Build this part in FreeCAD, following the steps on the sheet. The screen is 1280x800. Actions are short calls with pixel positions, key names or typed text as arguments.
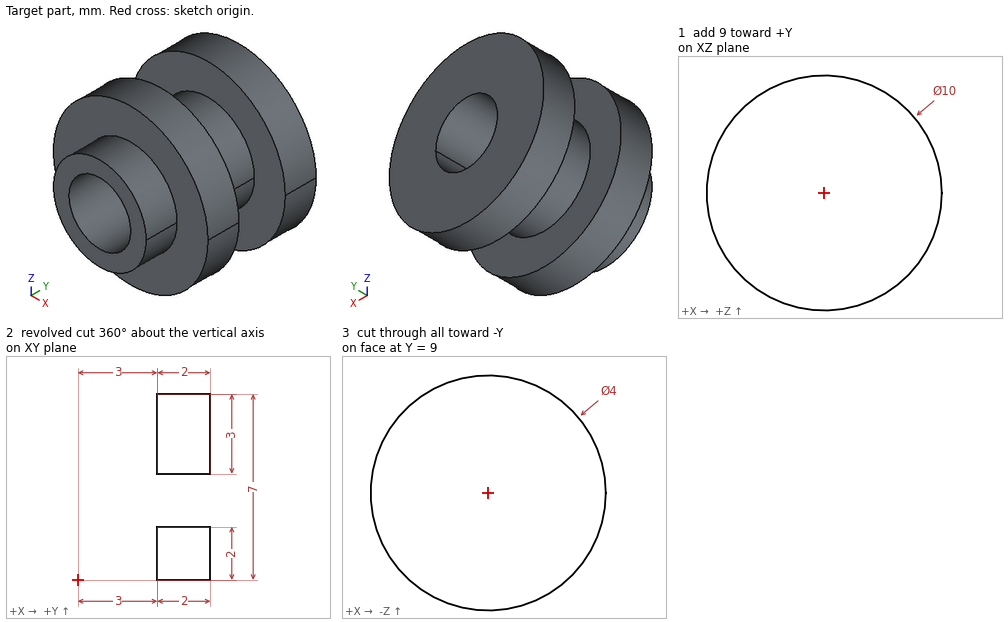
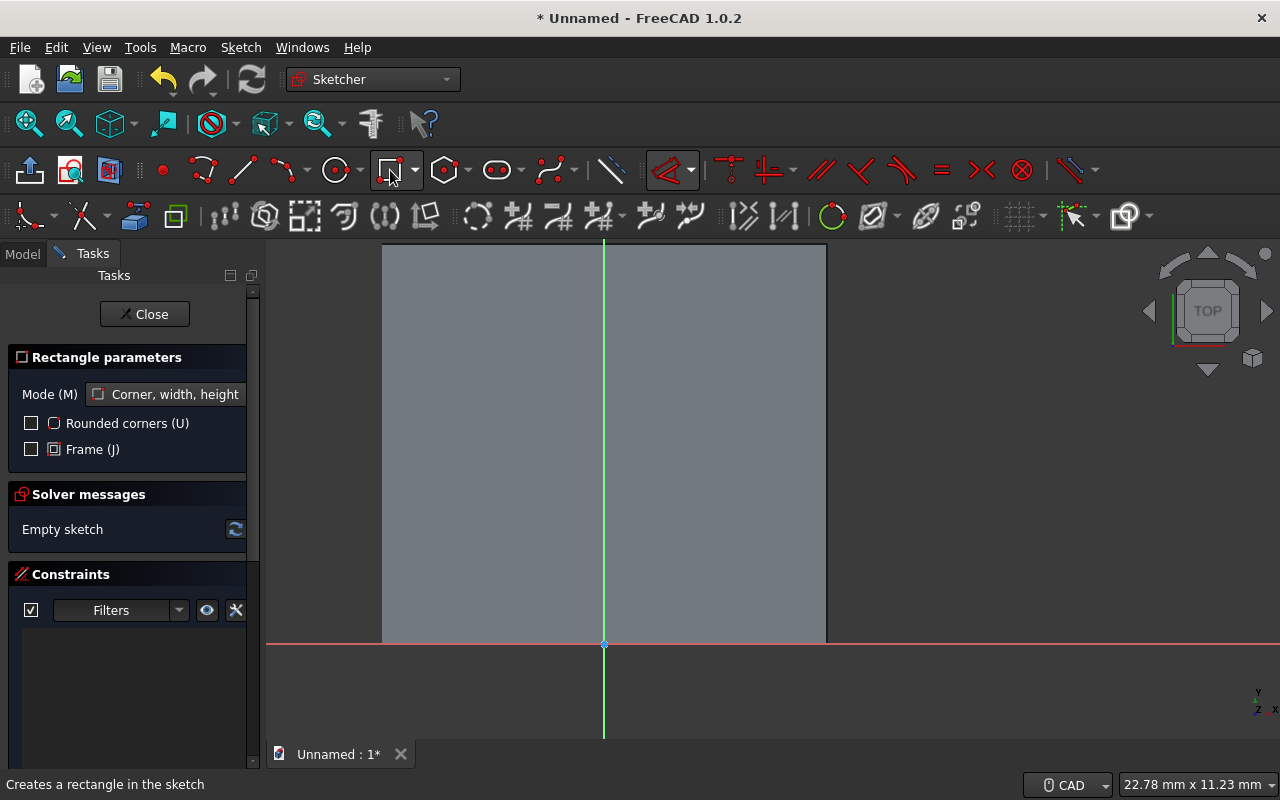
click(738, 333)
move(827, 466)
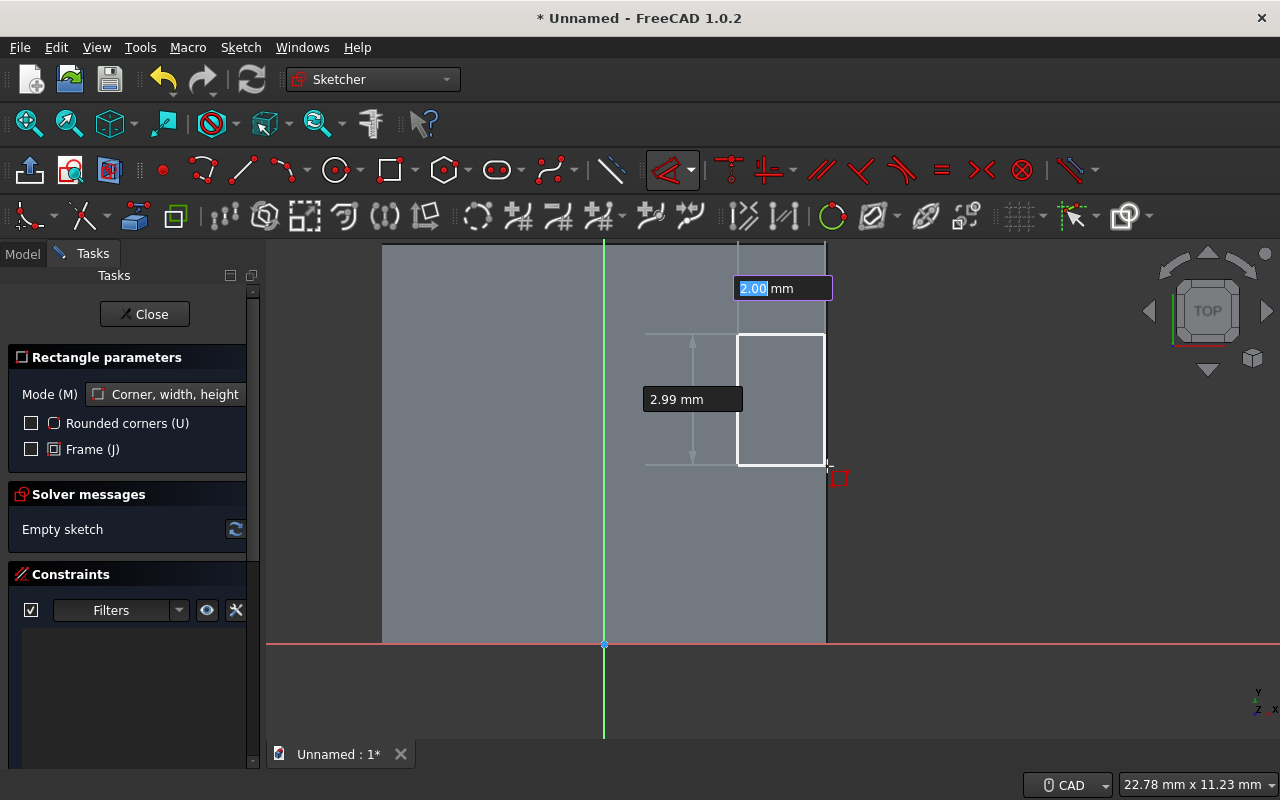
text(2)
key(Tab)
text(3)
key(Return)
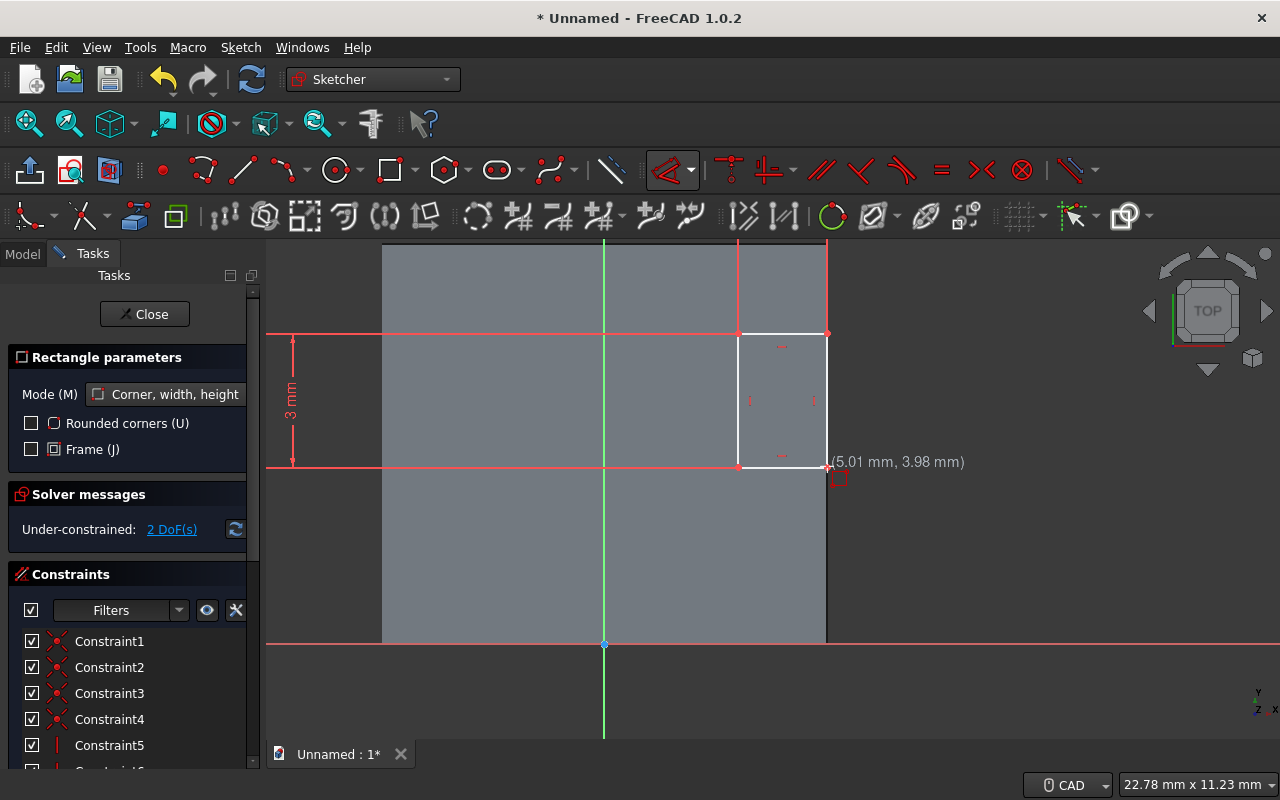
click(738, 555)
click(827, 644)
key(Escape)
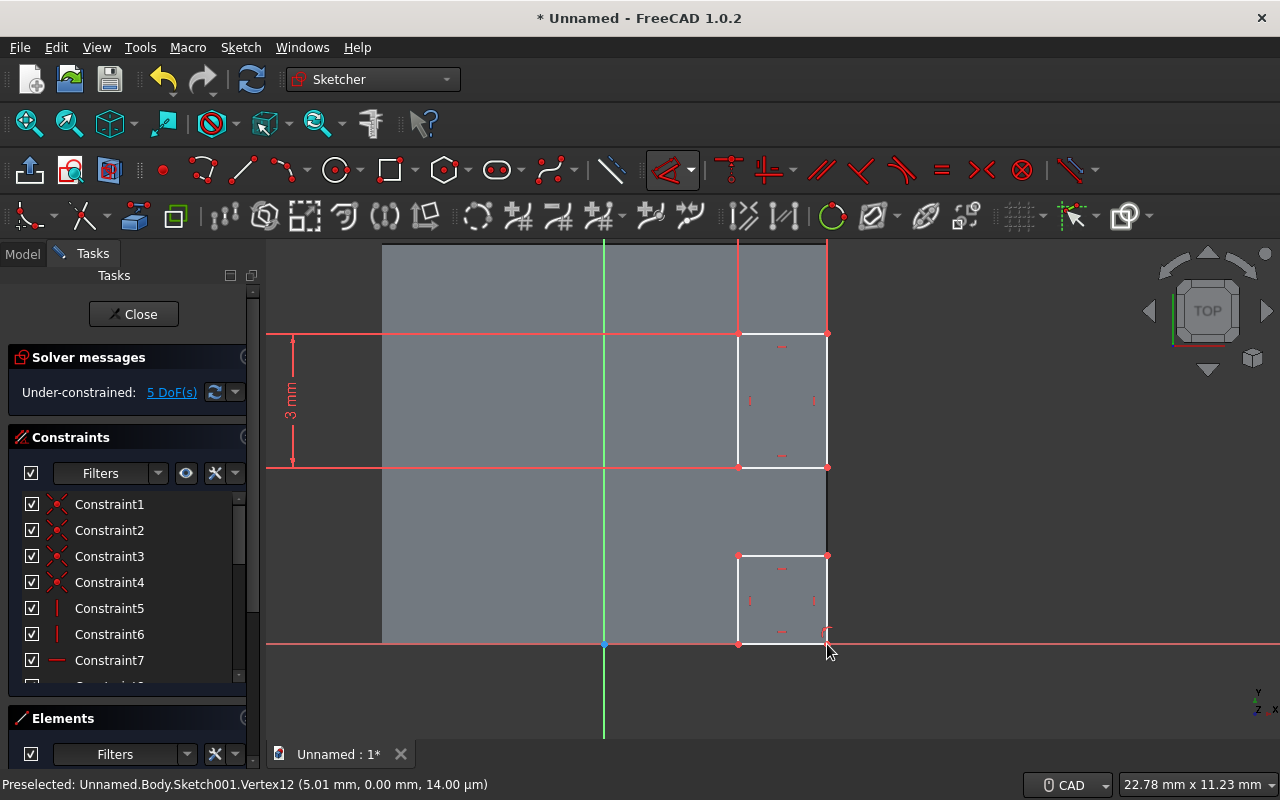
click(738, 582)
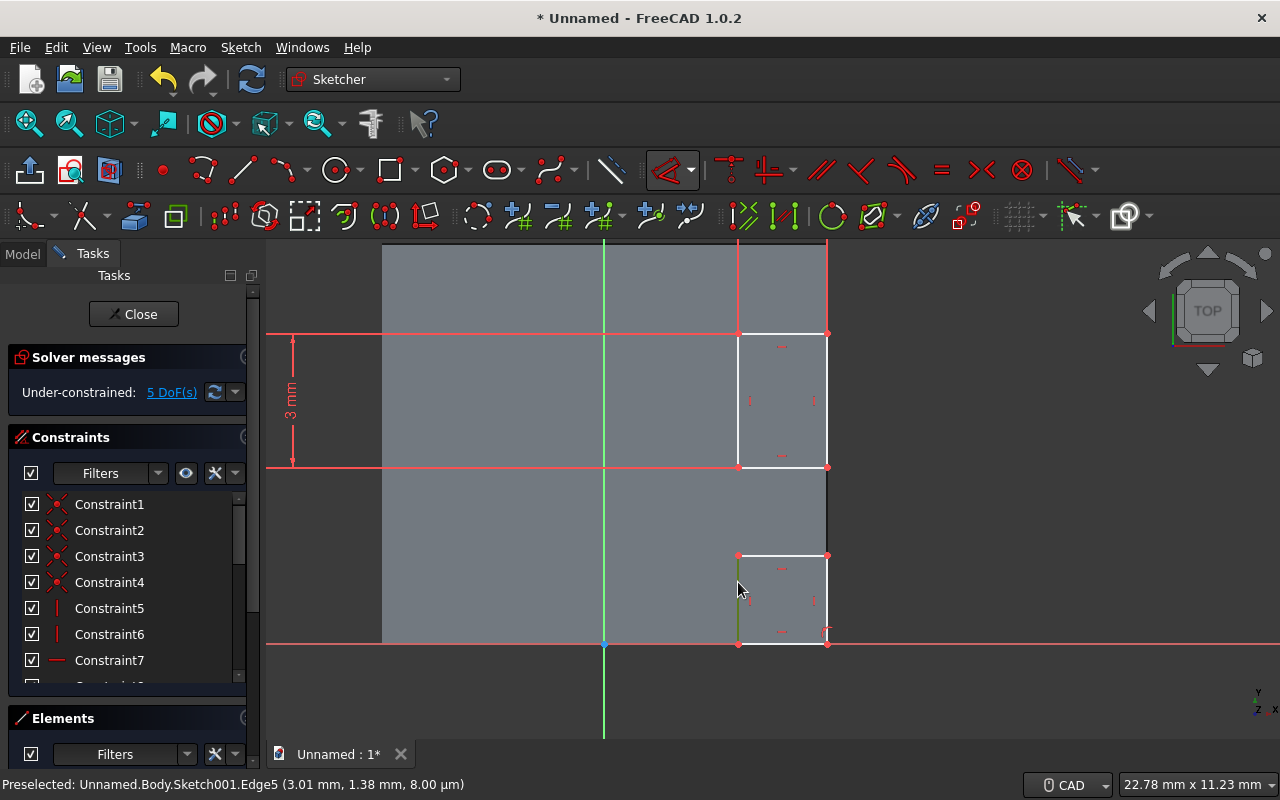
click(694, 170)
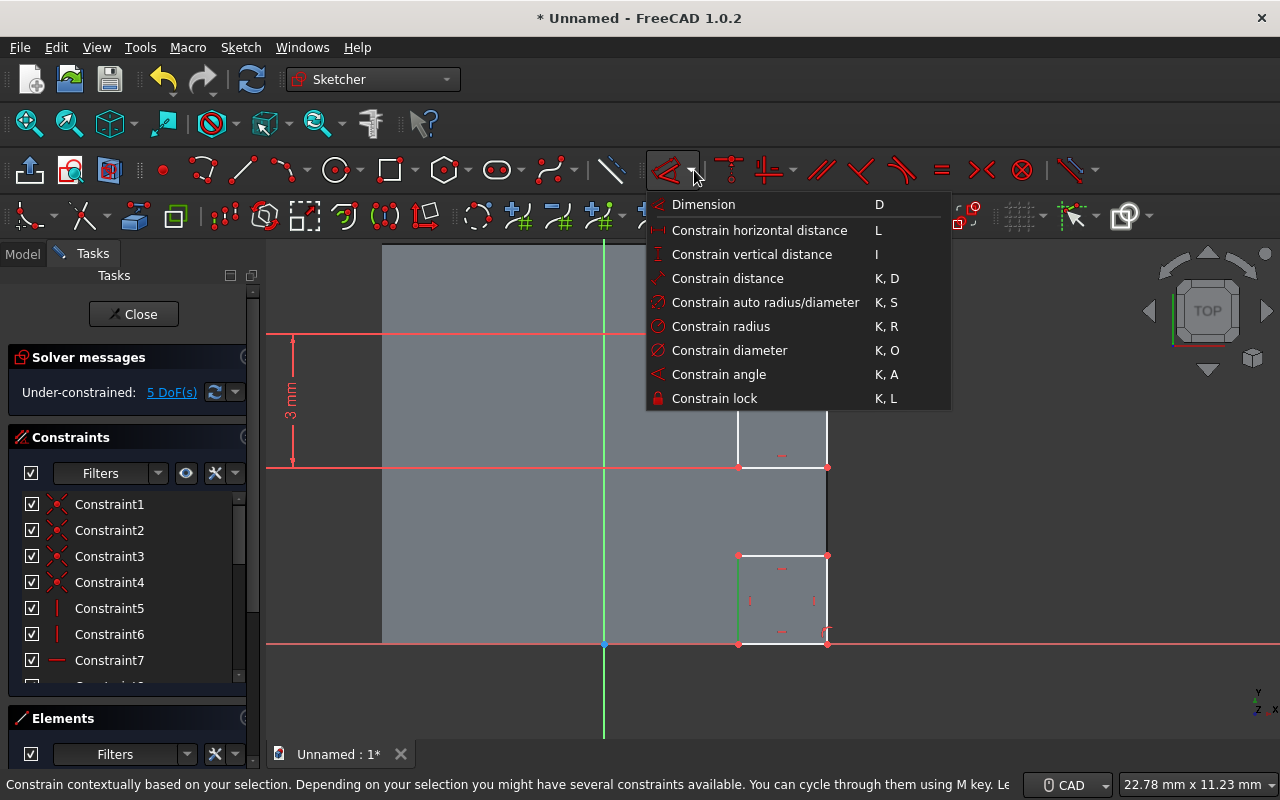
click(799, 254)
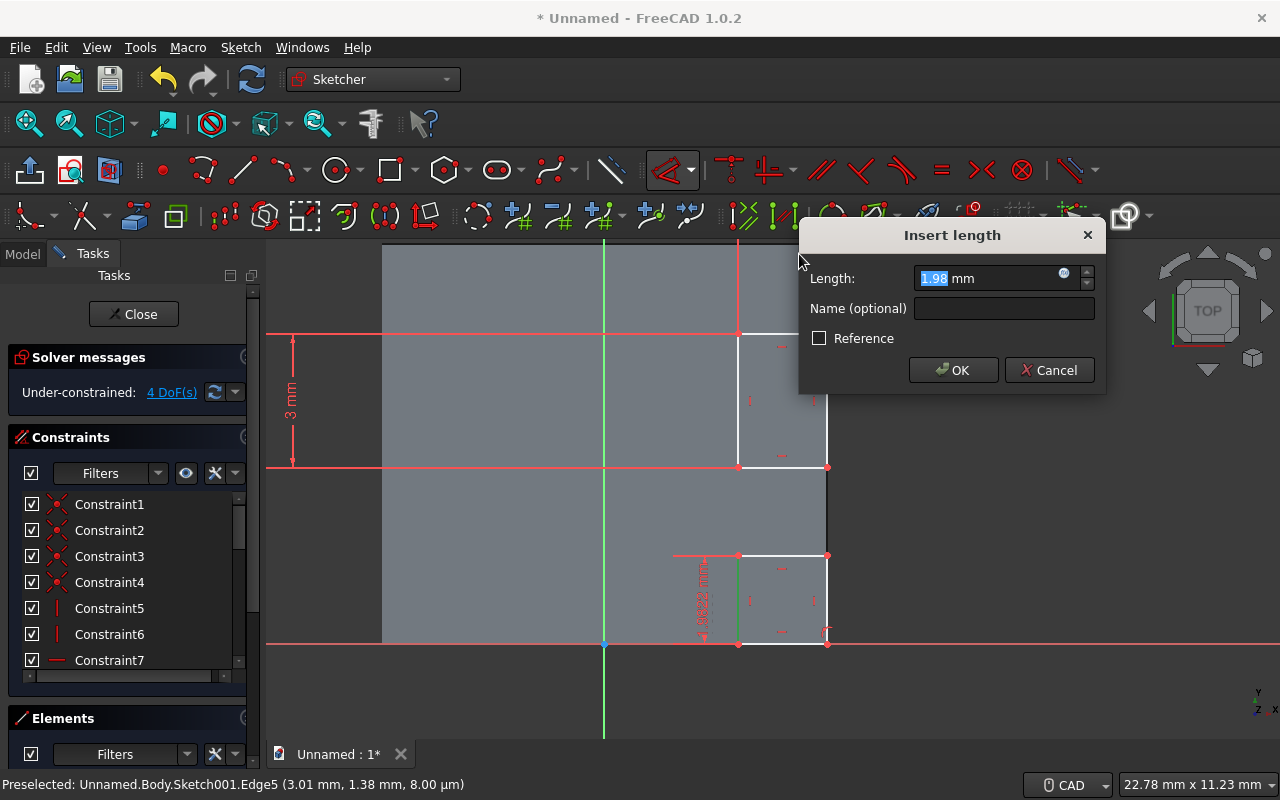
text(2)
key(Return)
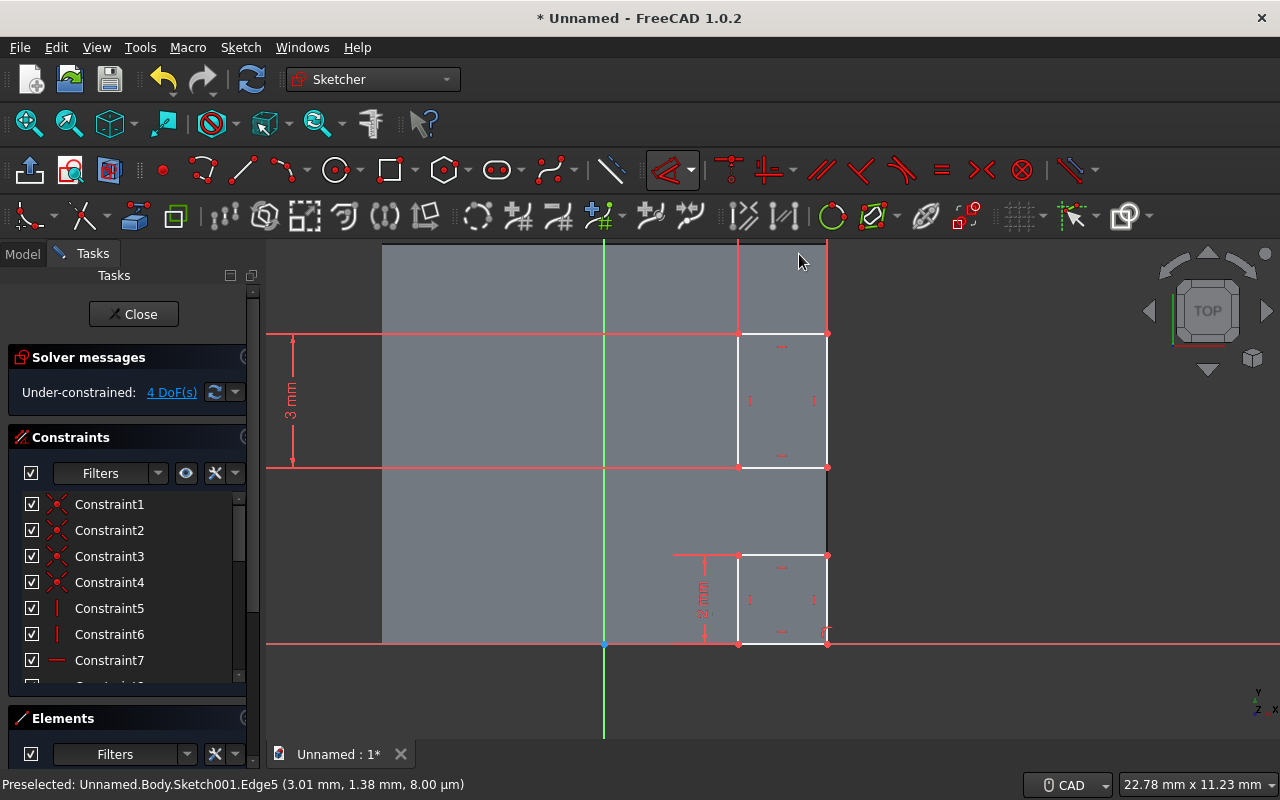
click(765, 644)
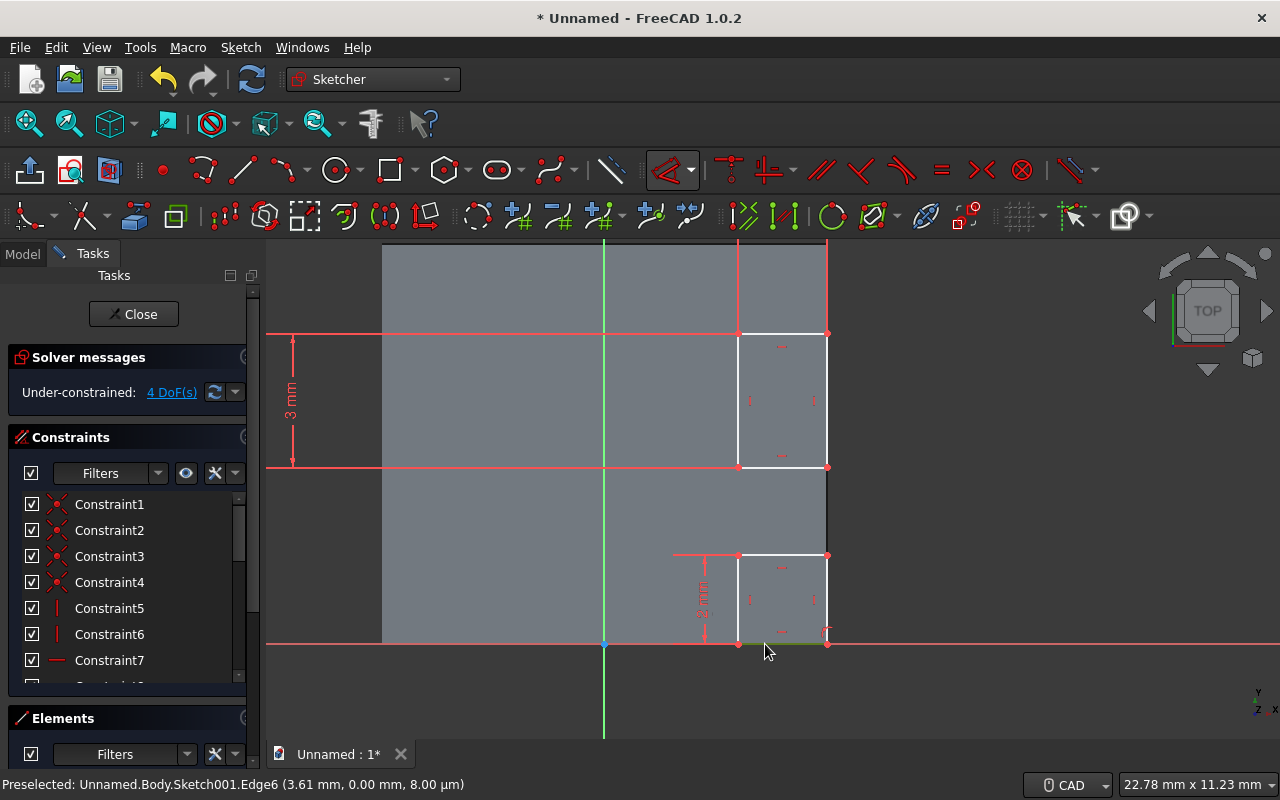
click(694, 170)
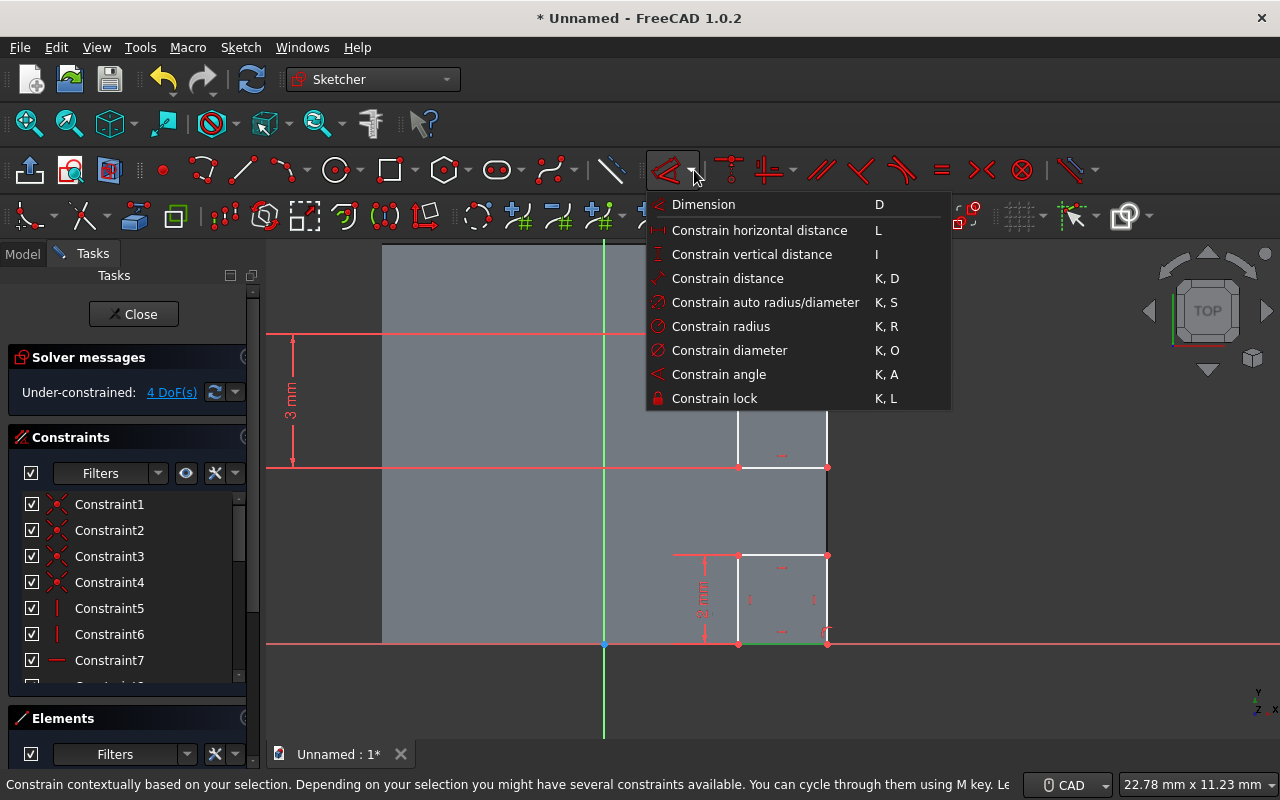
click(799, 230)